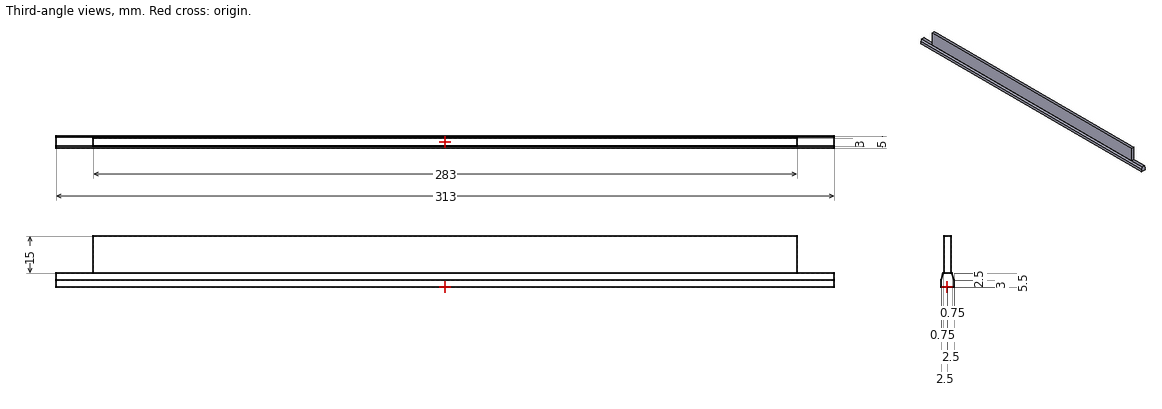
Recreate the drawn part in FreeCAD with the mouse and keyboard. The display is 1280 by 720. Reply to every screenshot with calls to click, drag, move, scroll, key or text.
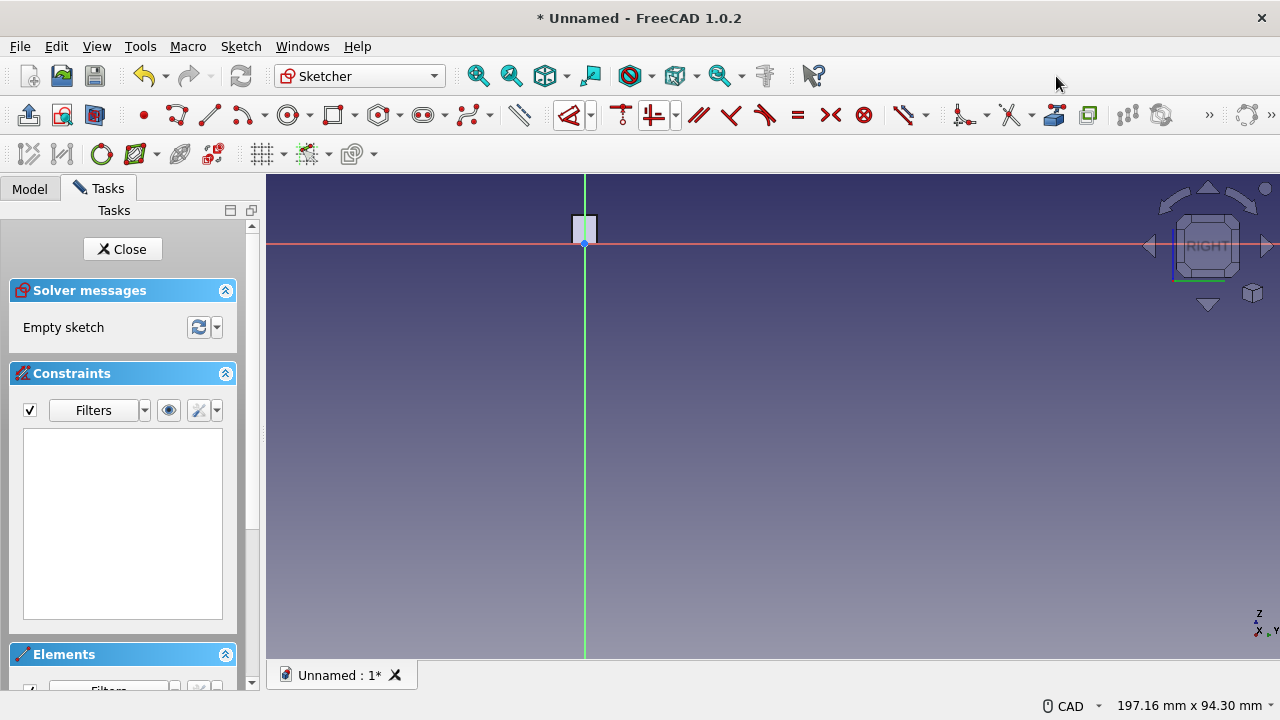
scroll(573, 211, up, 12)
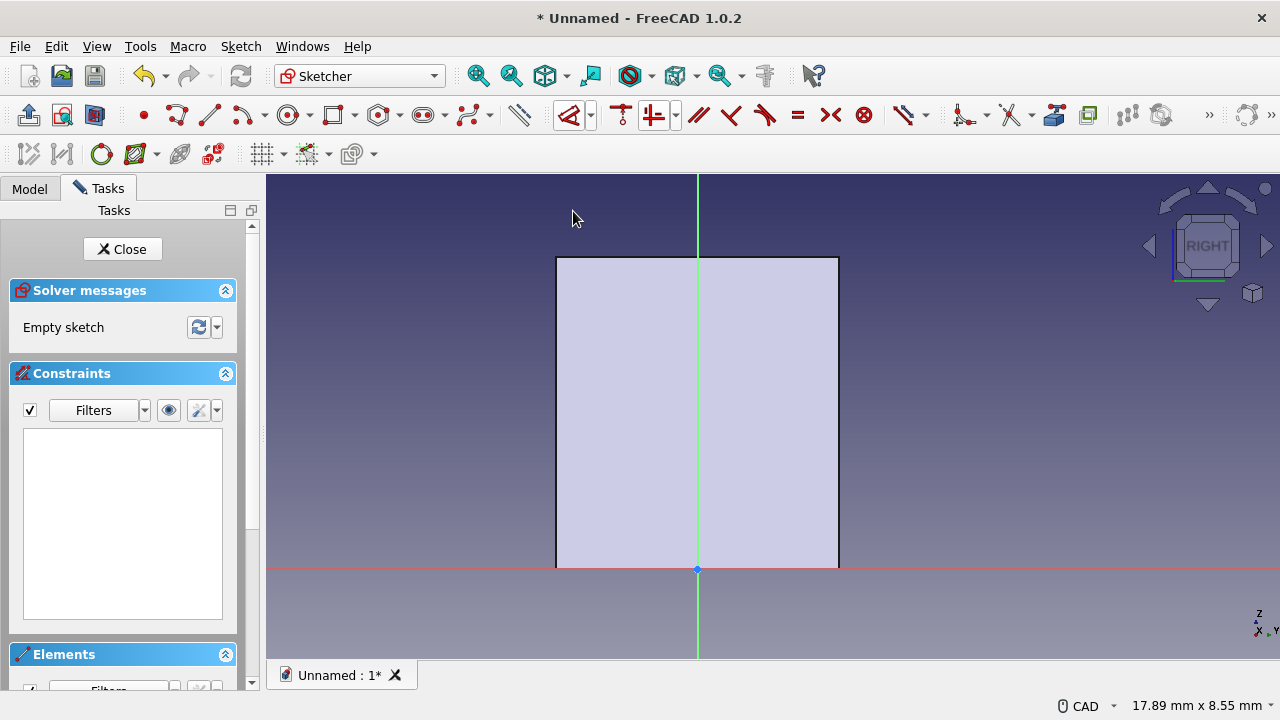
click(177, 116)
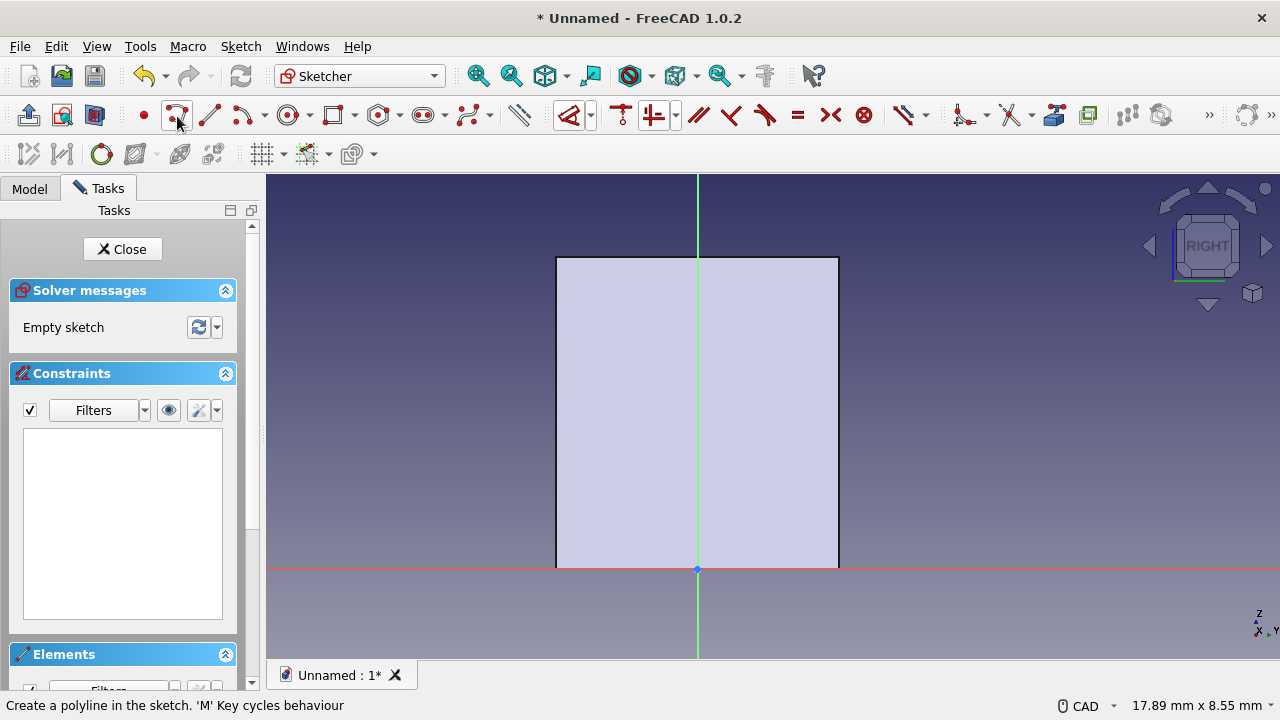
click(839, 399)
click(839, 257)
click(797, 257)
click(839, 400)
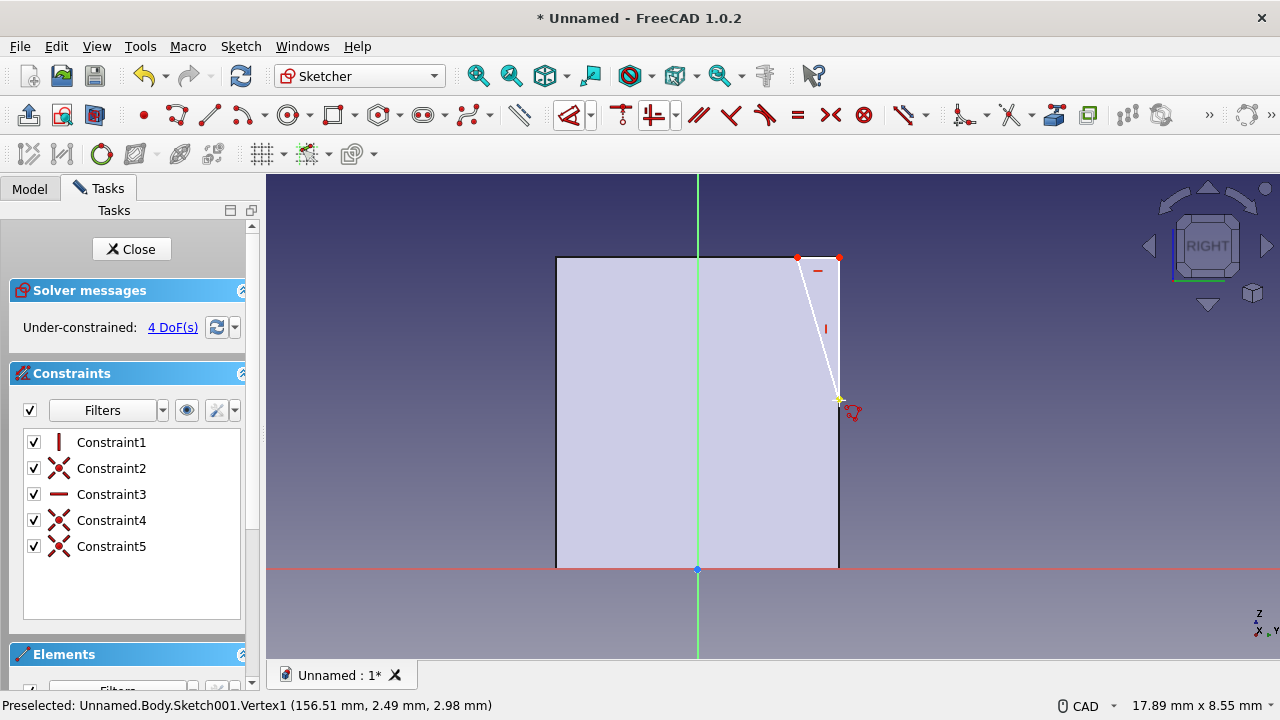
click(556, 399)
click(599, 257)
click(556, 257)
click(556, 400)
key(Escape)
key(Escape)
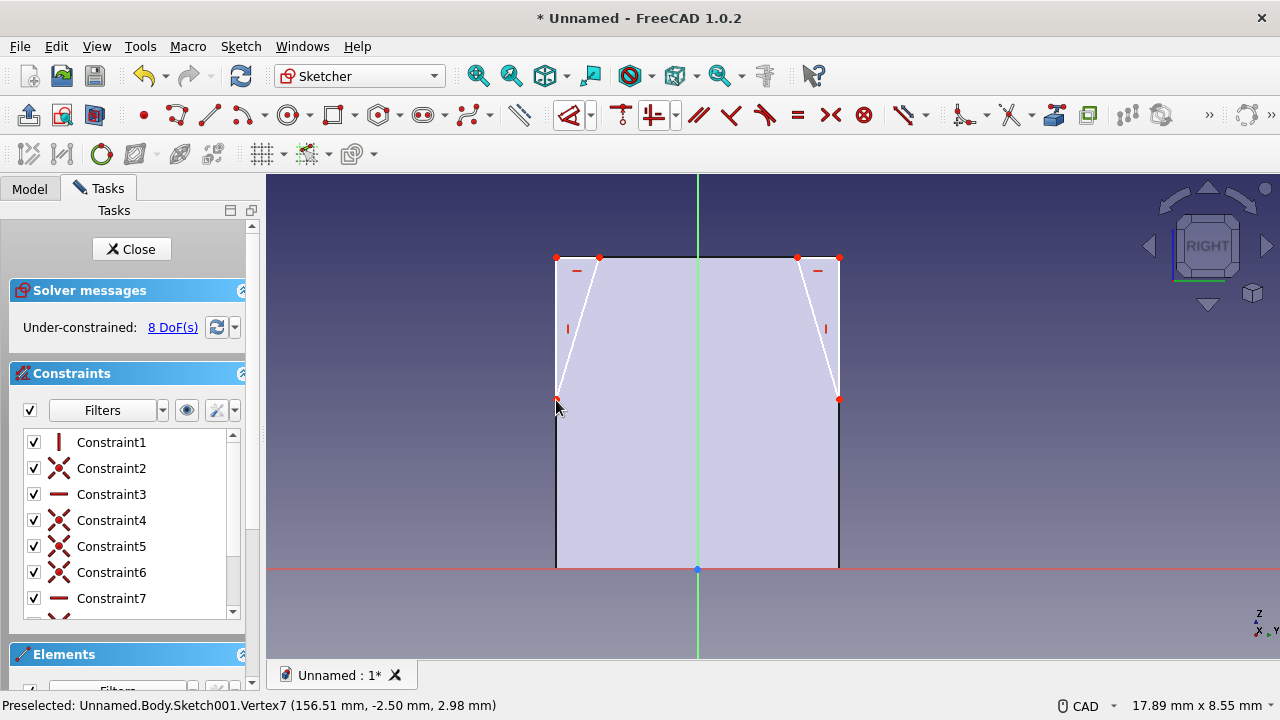
click(568, 116)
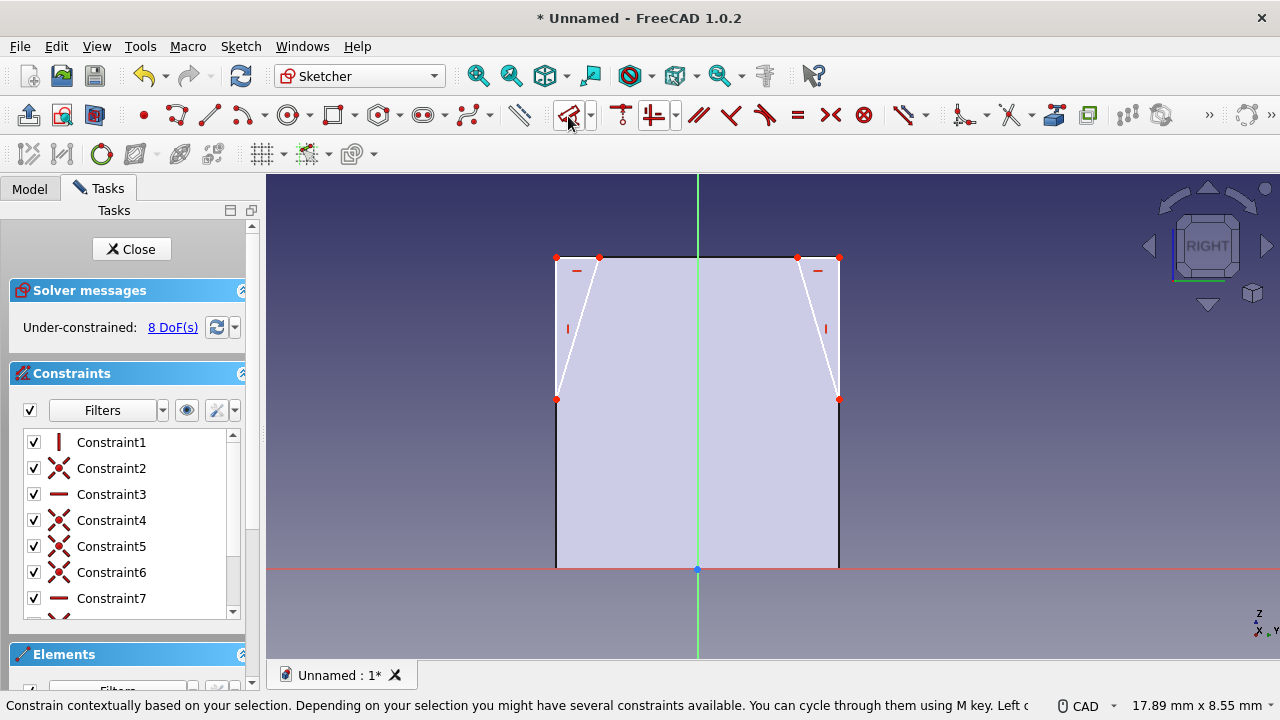
click(839, 400)
click(873, 485)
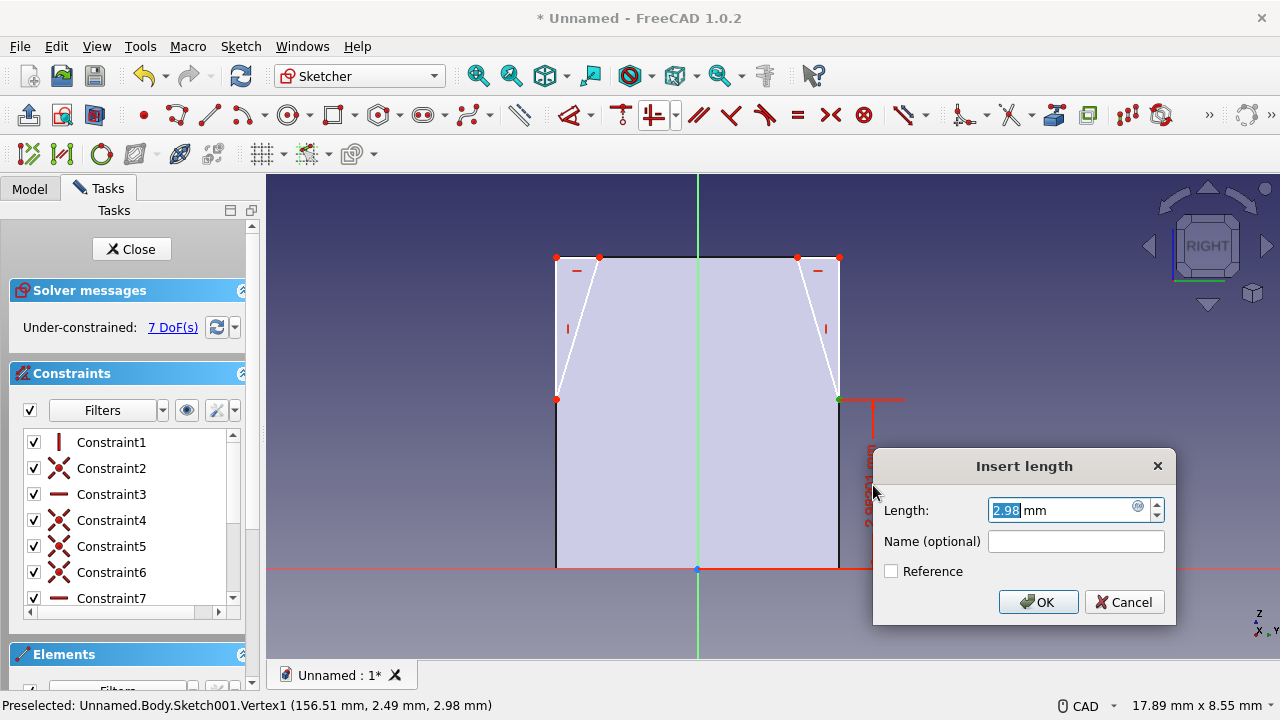
text(3)
key(Return)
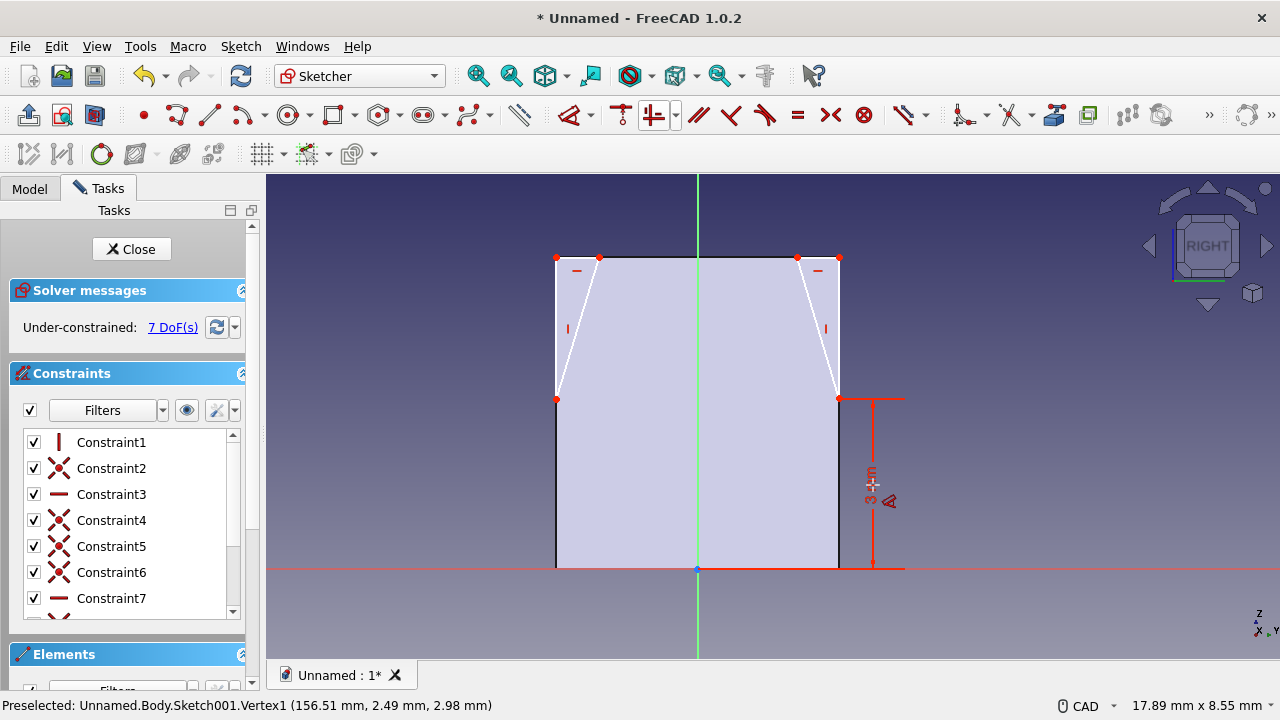
click(556, 400)
click(522, 485)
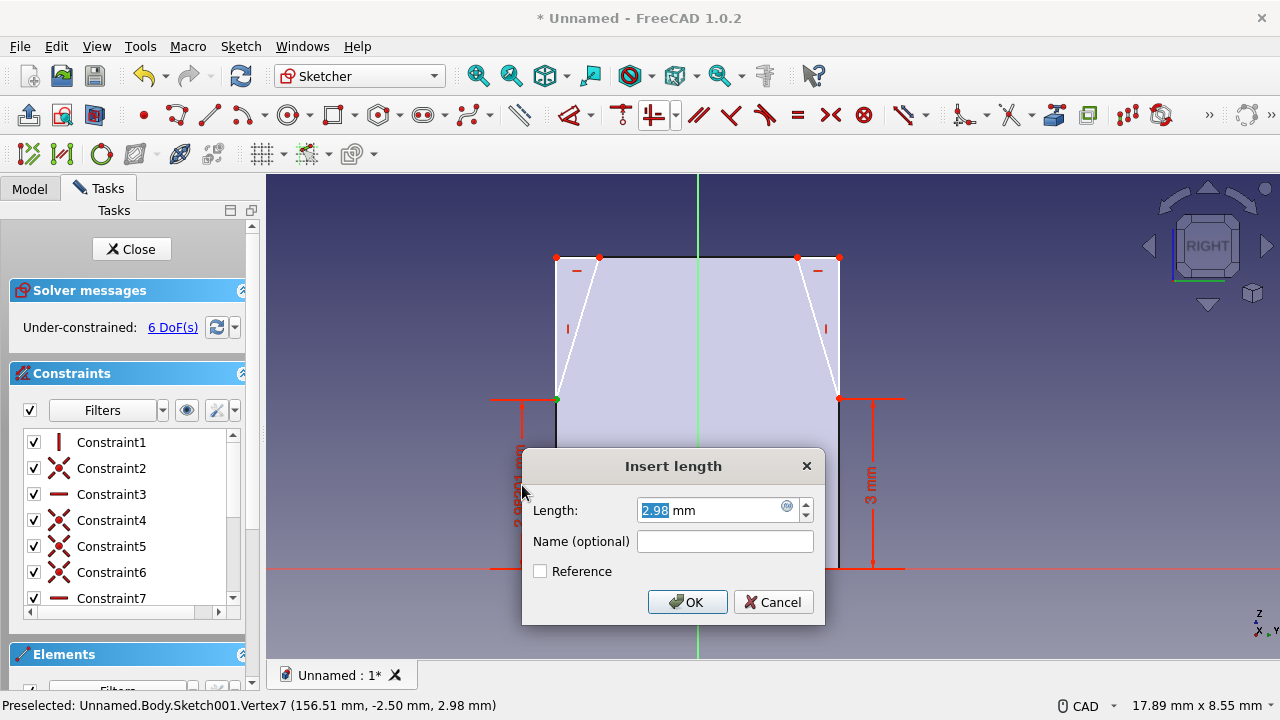
text(3)
key(Return)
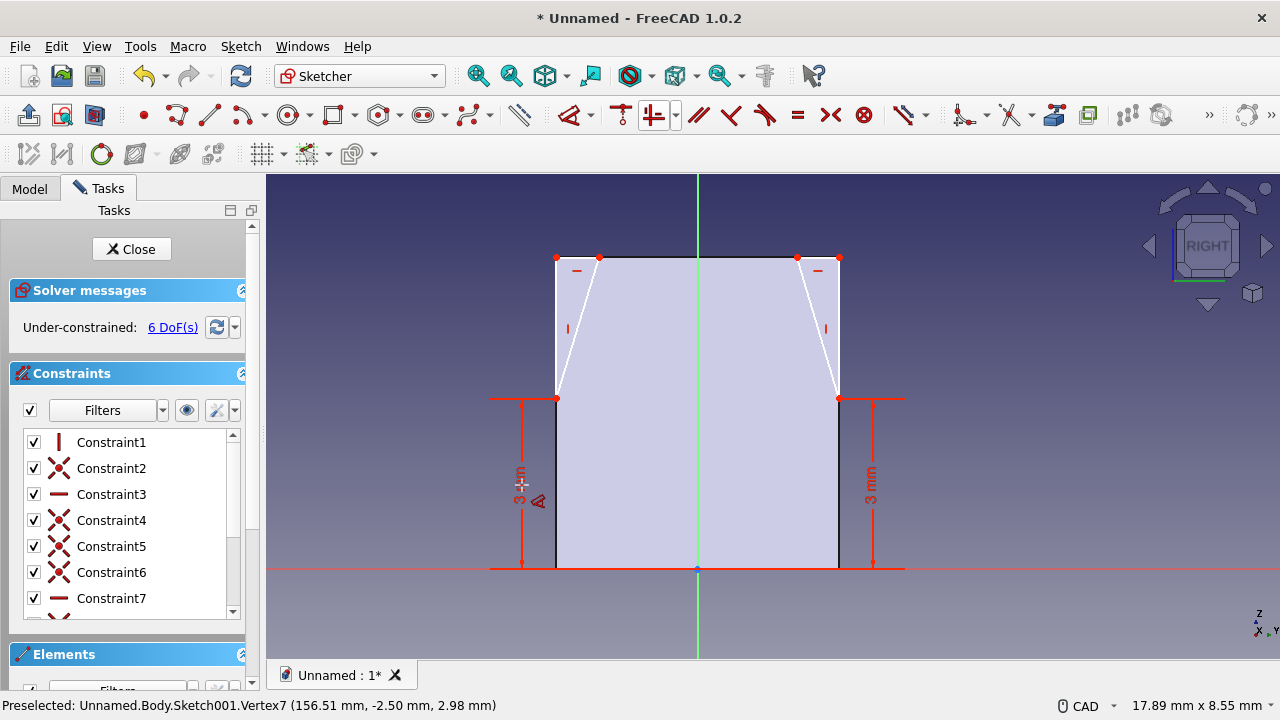
click(839, 357)
click(873, 328)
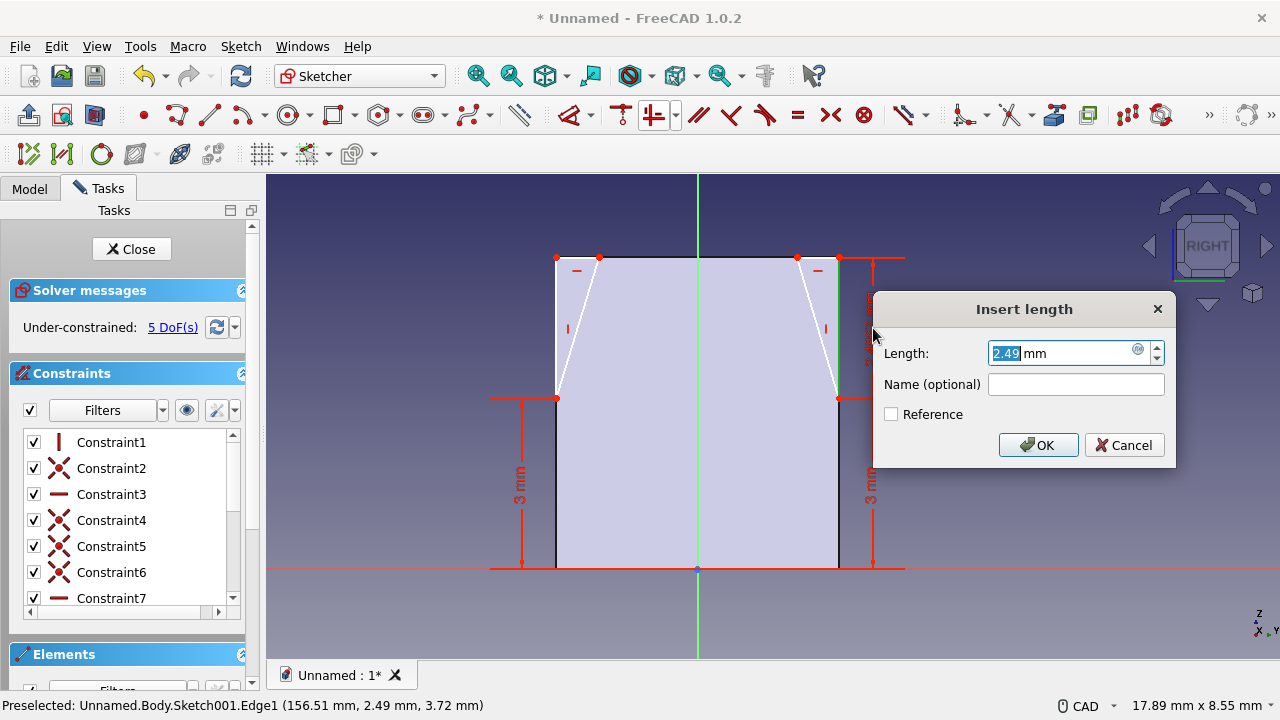
text(2.5)
key(Return)